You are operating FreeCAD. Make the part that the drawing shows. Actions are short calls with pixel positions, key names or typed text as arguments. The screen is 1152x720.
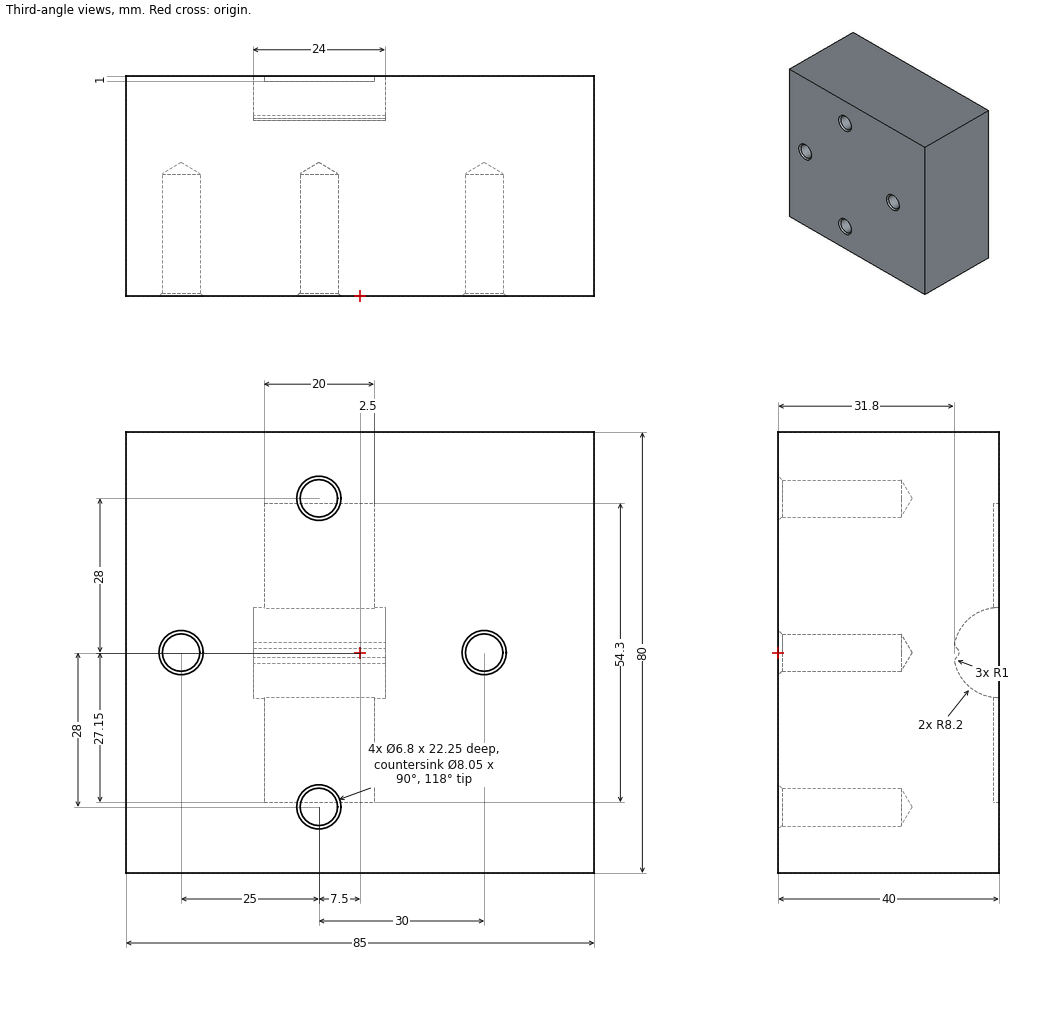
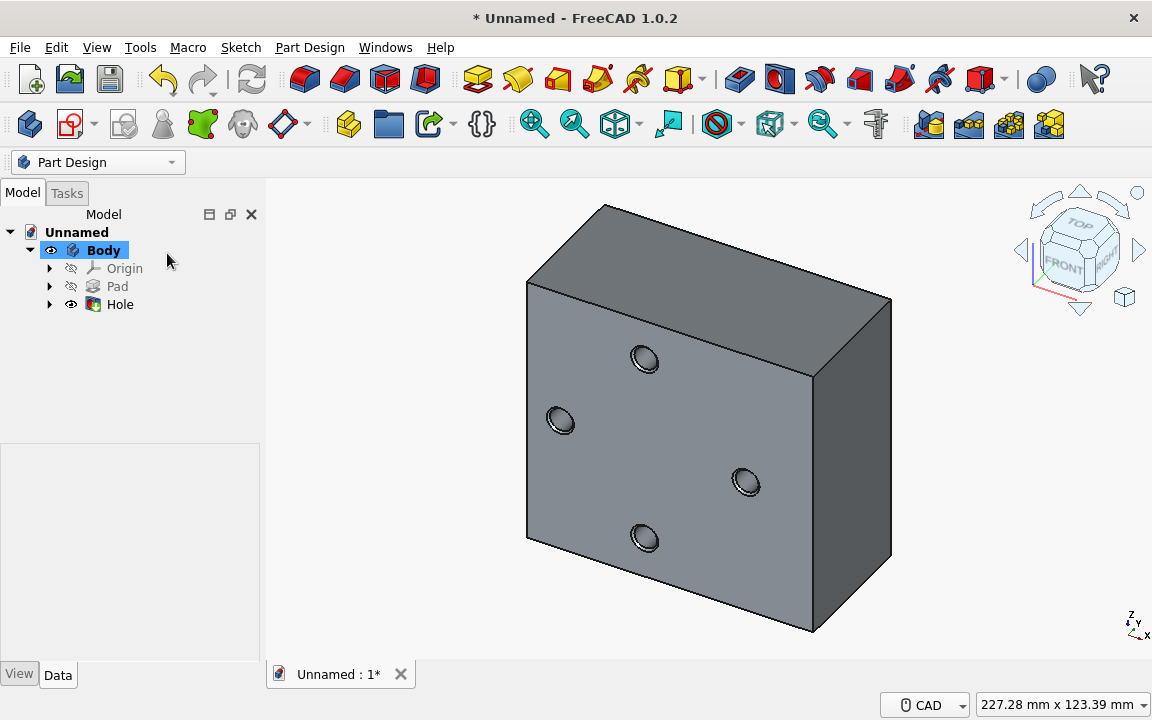
key(4)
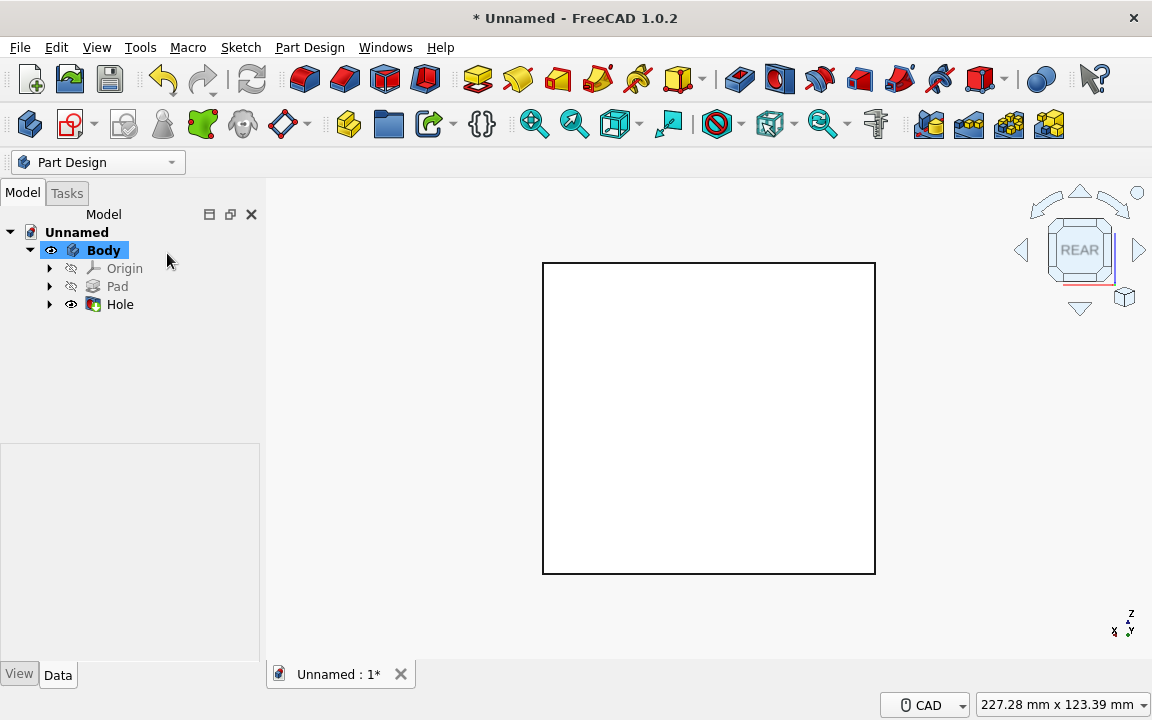
click(709, 418)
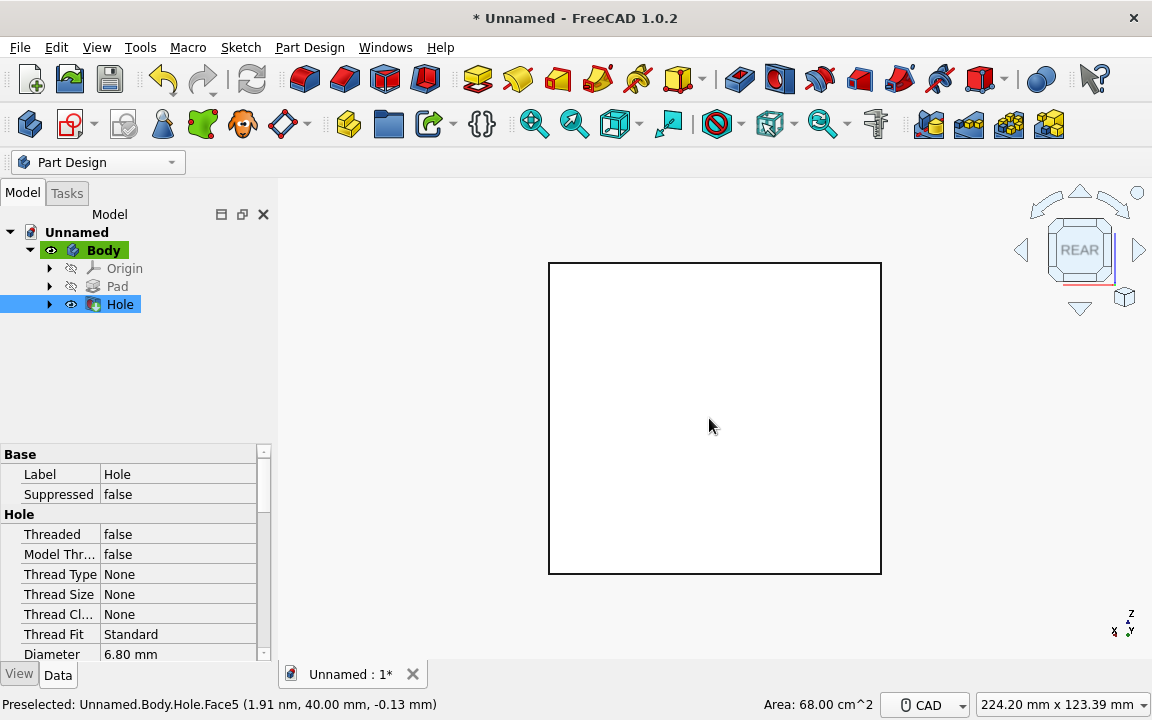
click(70, 124)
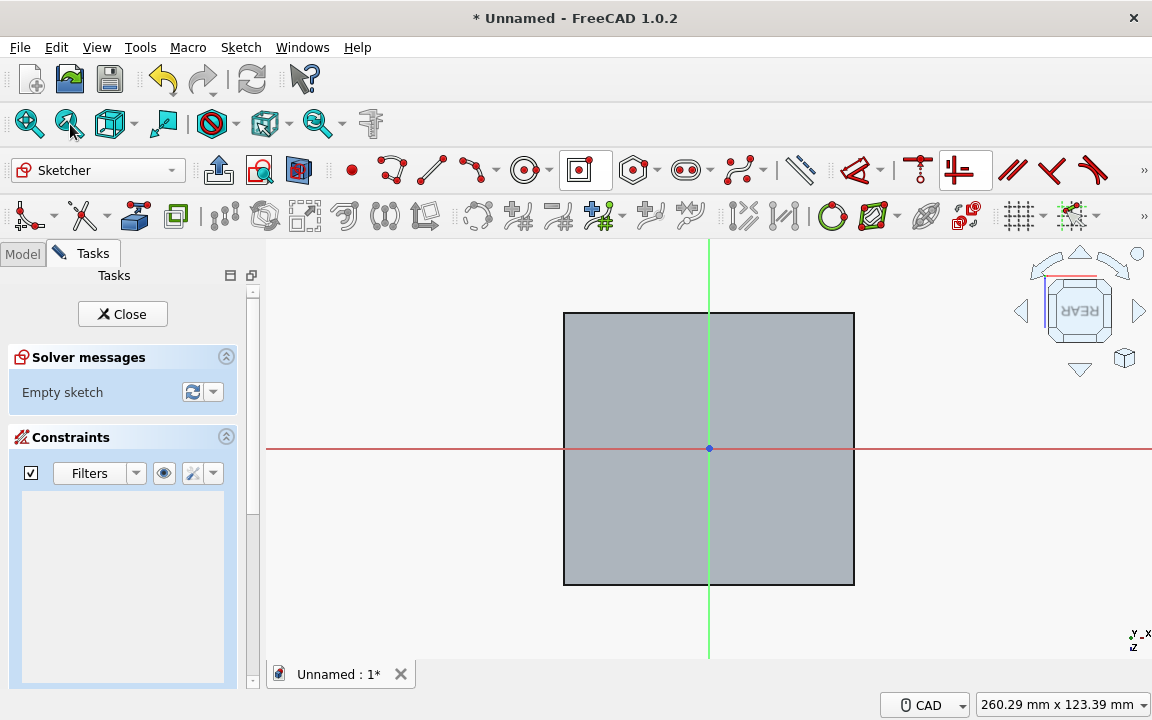
scroll(771, 449, up, 2)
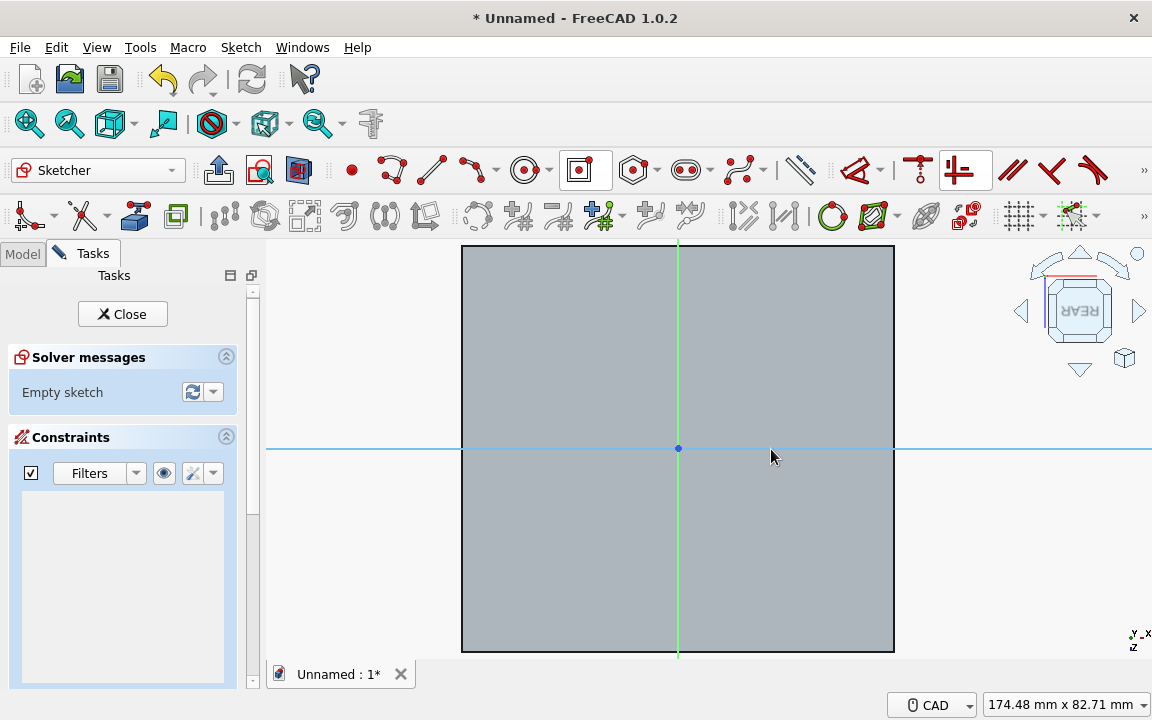
click(606, 170)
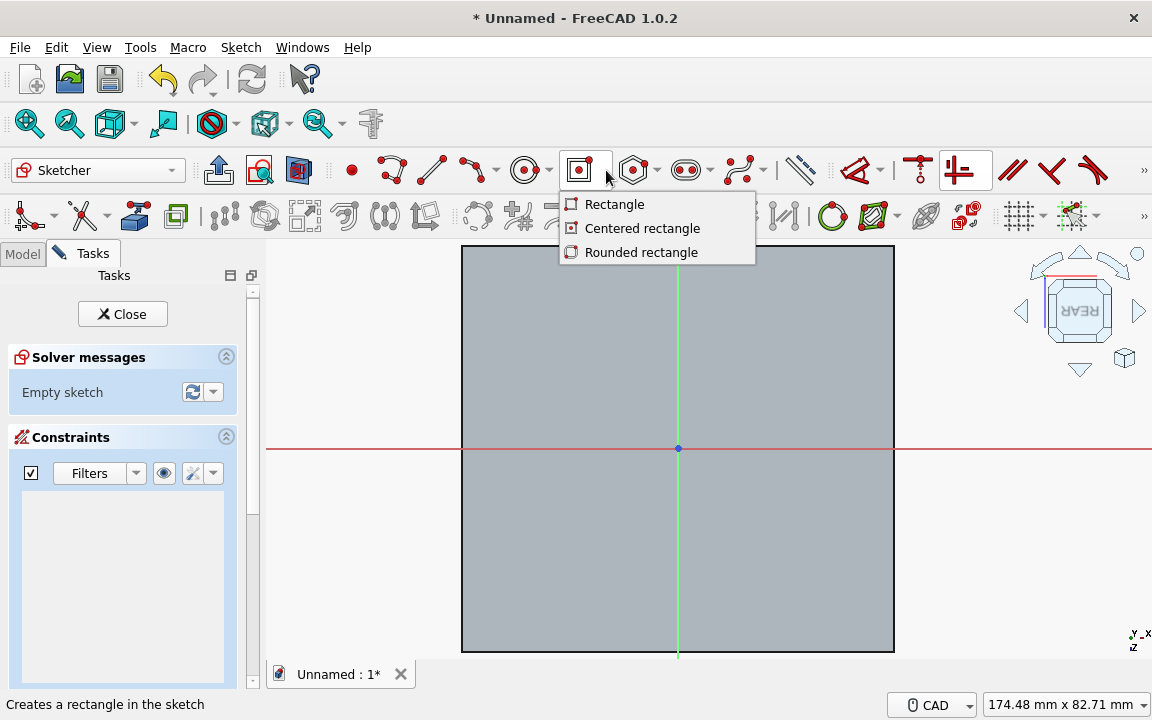
click(658, 204)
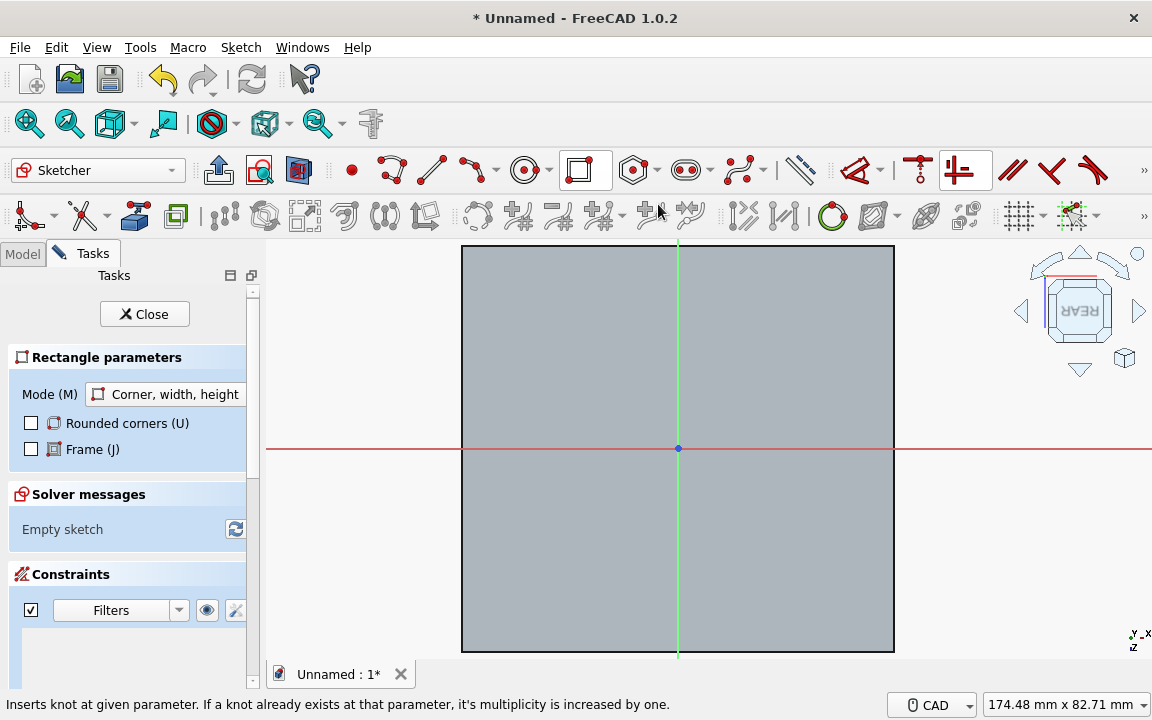
click(589, 311)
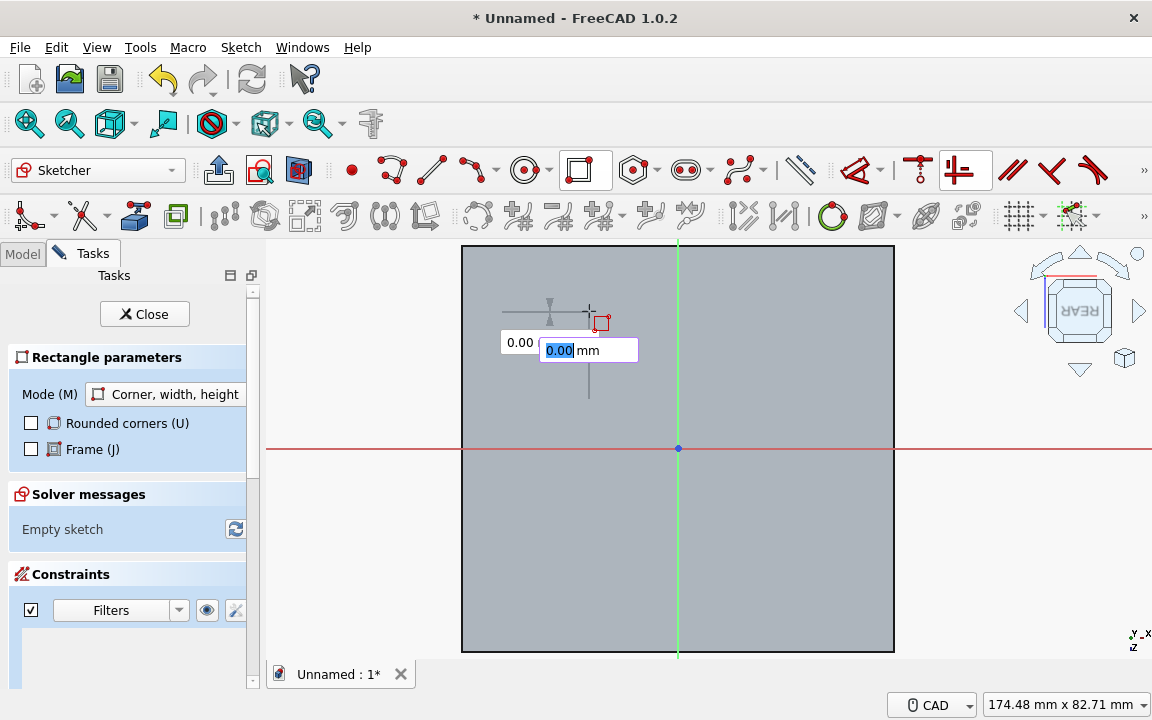
scroll(691, 587, up, 2)
move(691, 586)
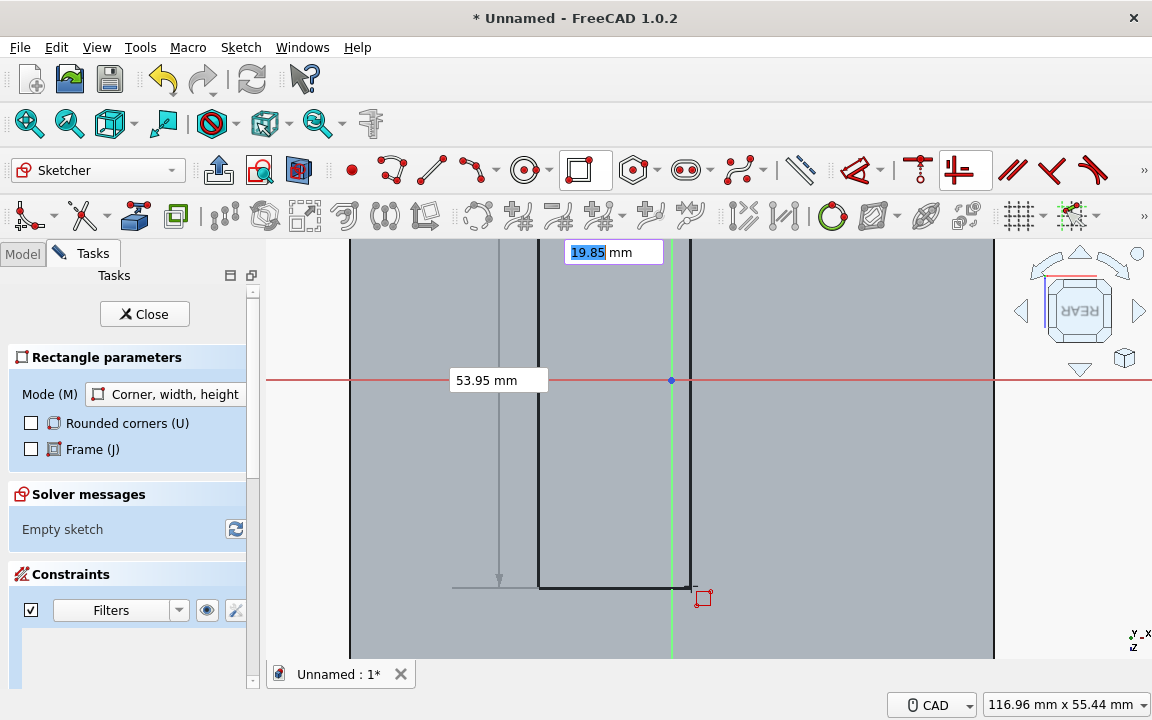
text(20)
key(Tab)
text(54.3)
key(Return)
key(Escape)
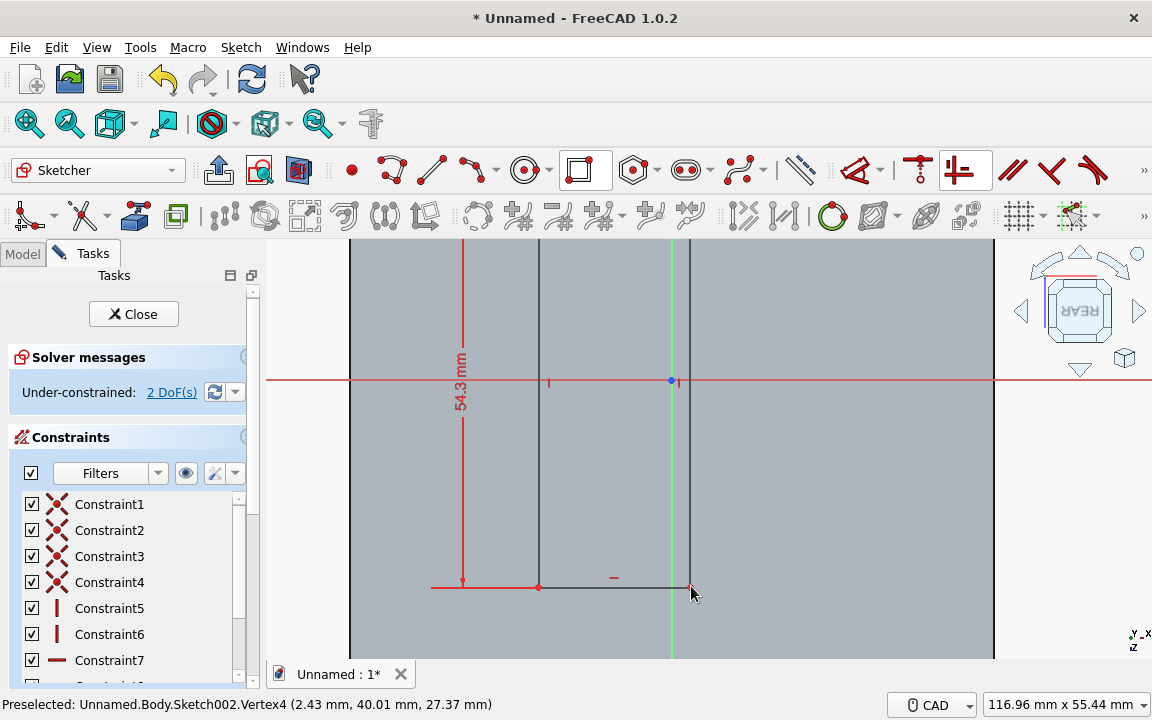
click(856, 170)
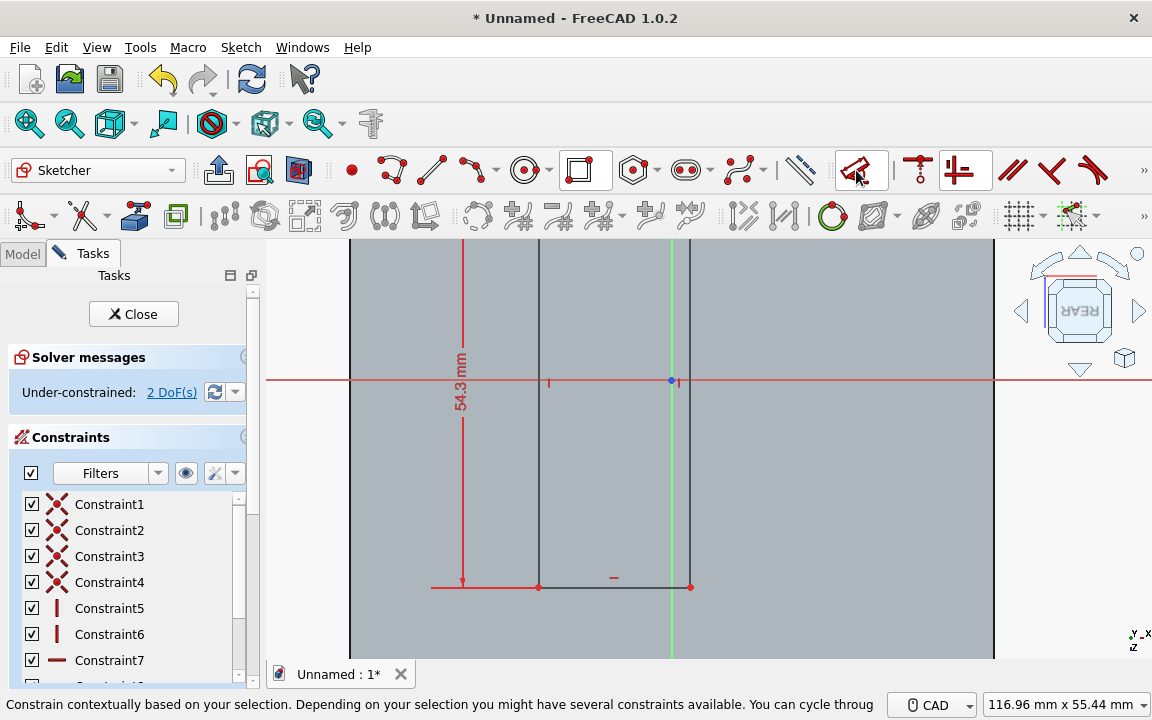
scroll(690, 588, up, 4)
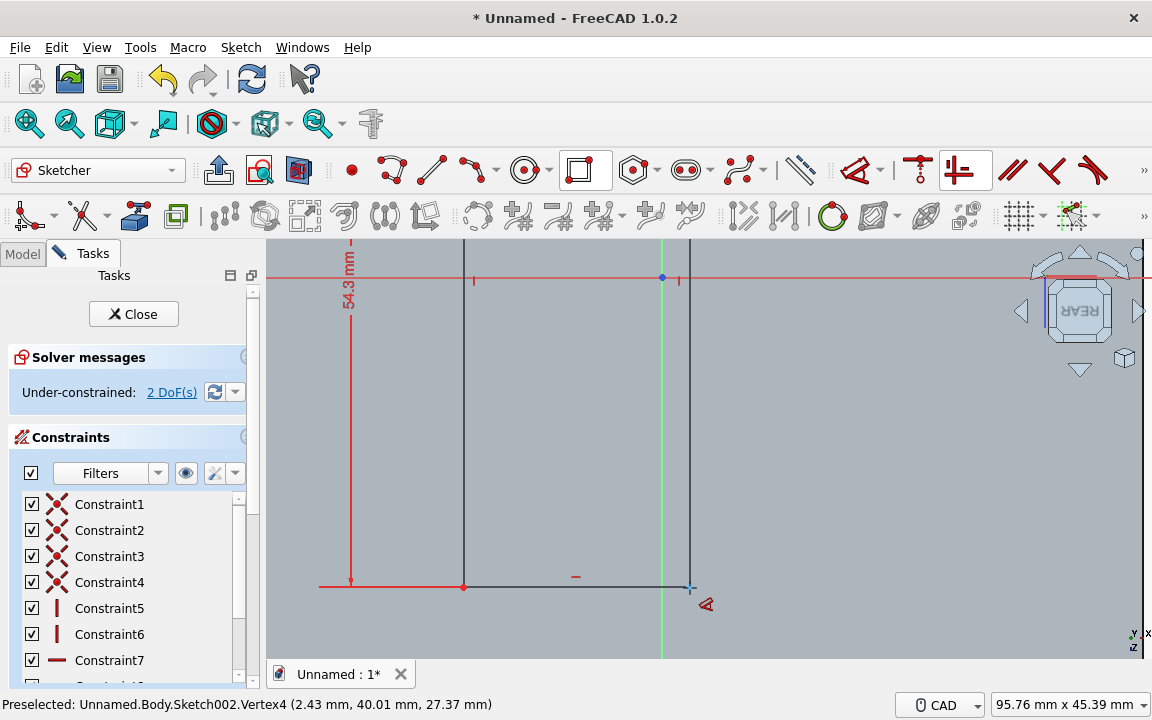
click(690, 586)
click(669, 620)